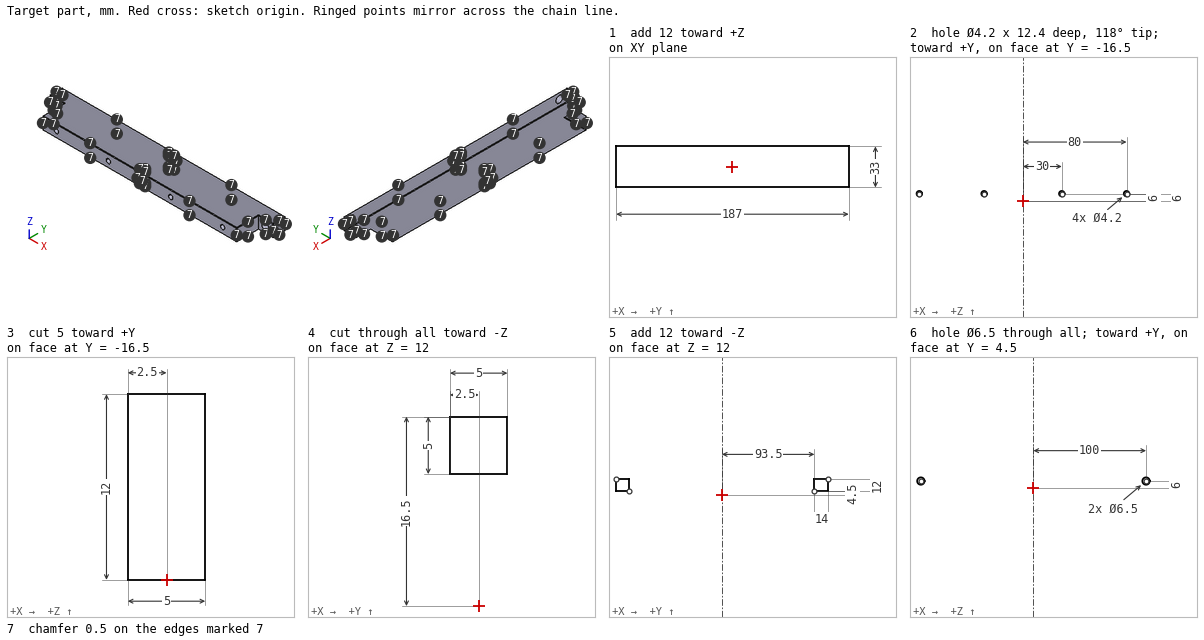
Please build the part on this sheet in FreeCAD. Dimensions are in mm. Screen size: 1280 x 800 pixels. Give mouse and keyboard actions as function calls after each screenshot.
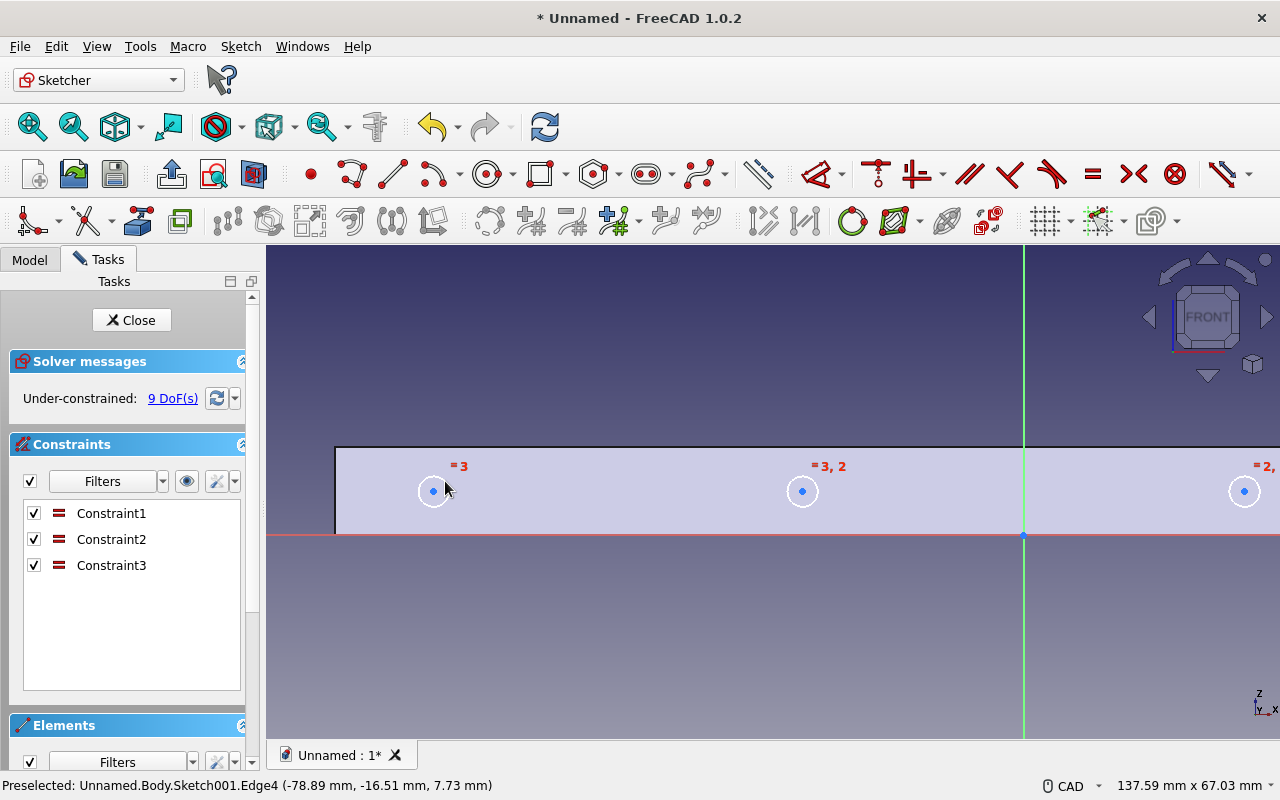
scroll(444, 481, down, 4)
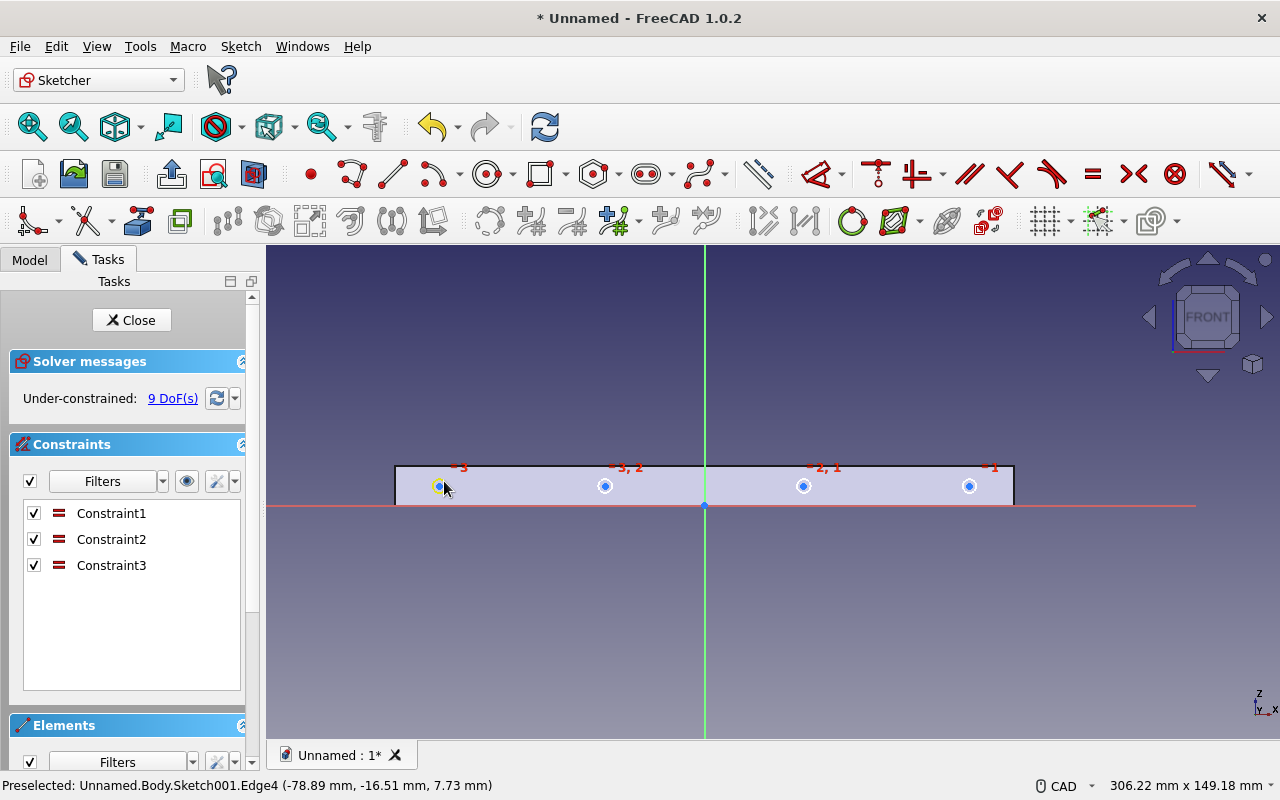
click(804, 486)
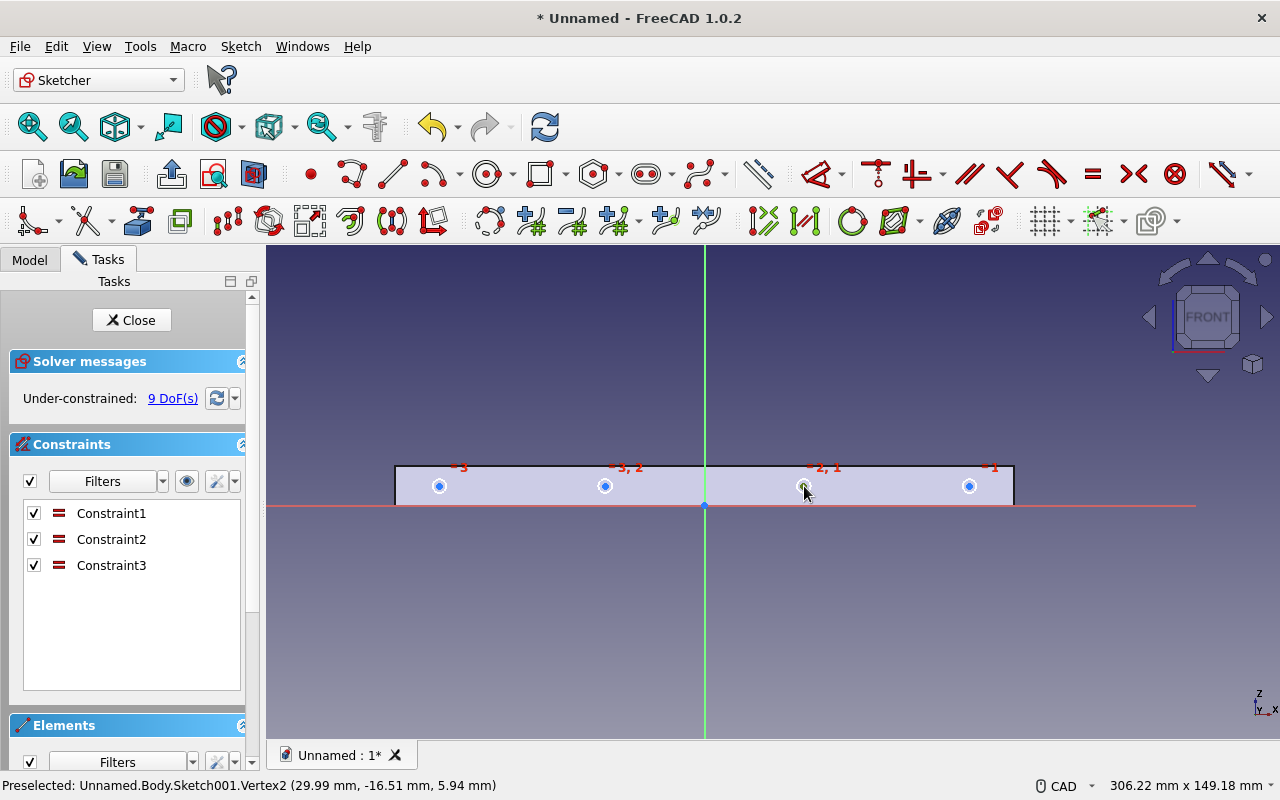
click(605, 486)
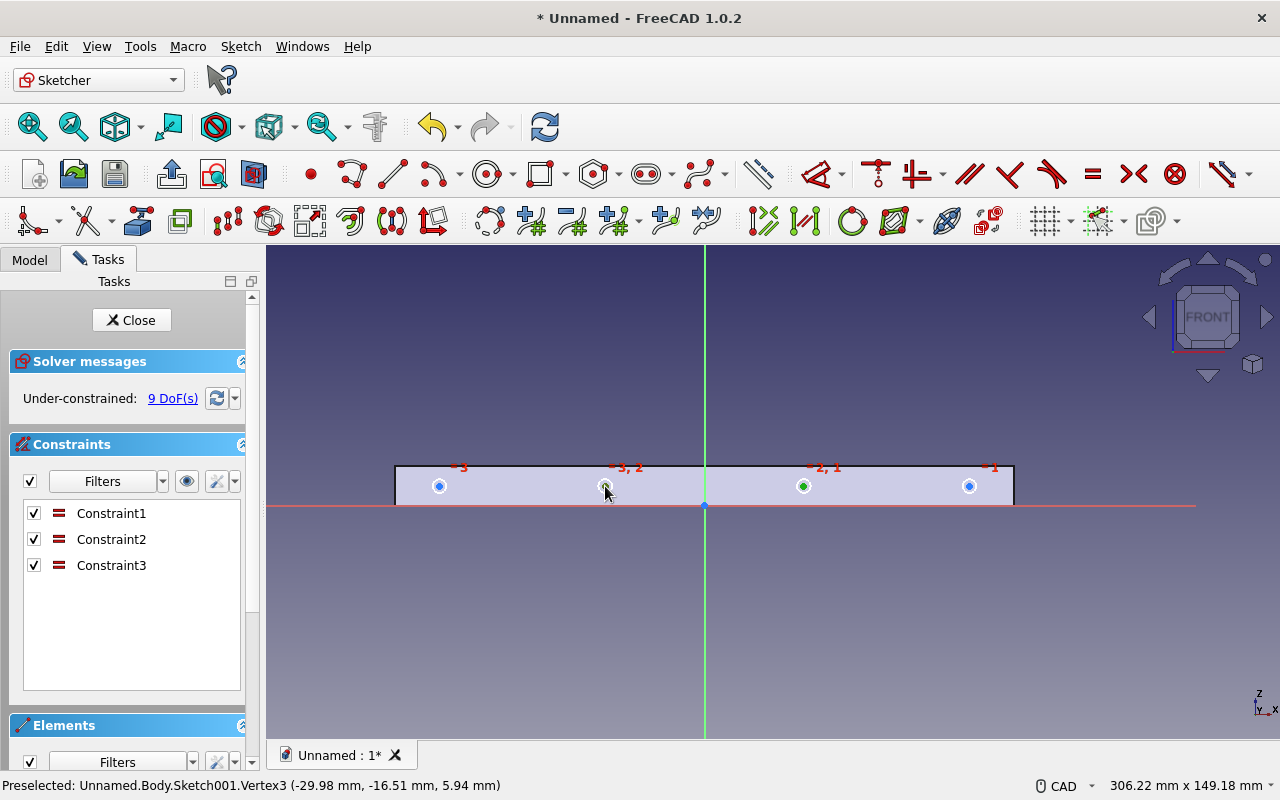
click(705, 680)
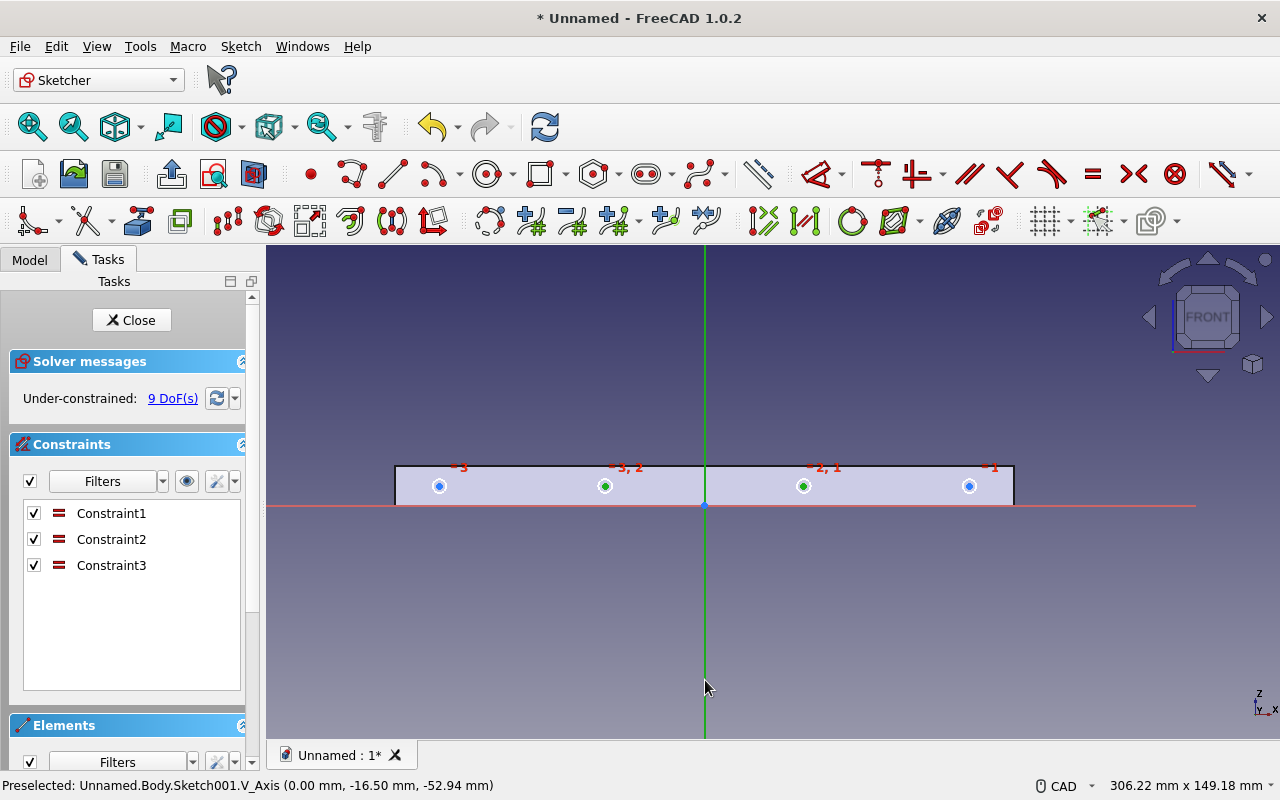
key(s)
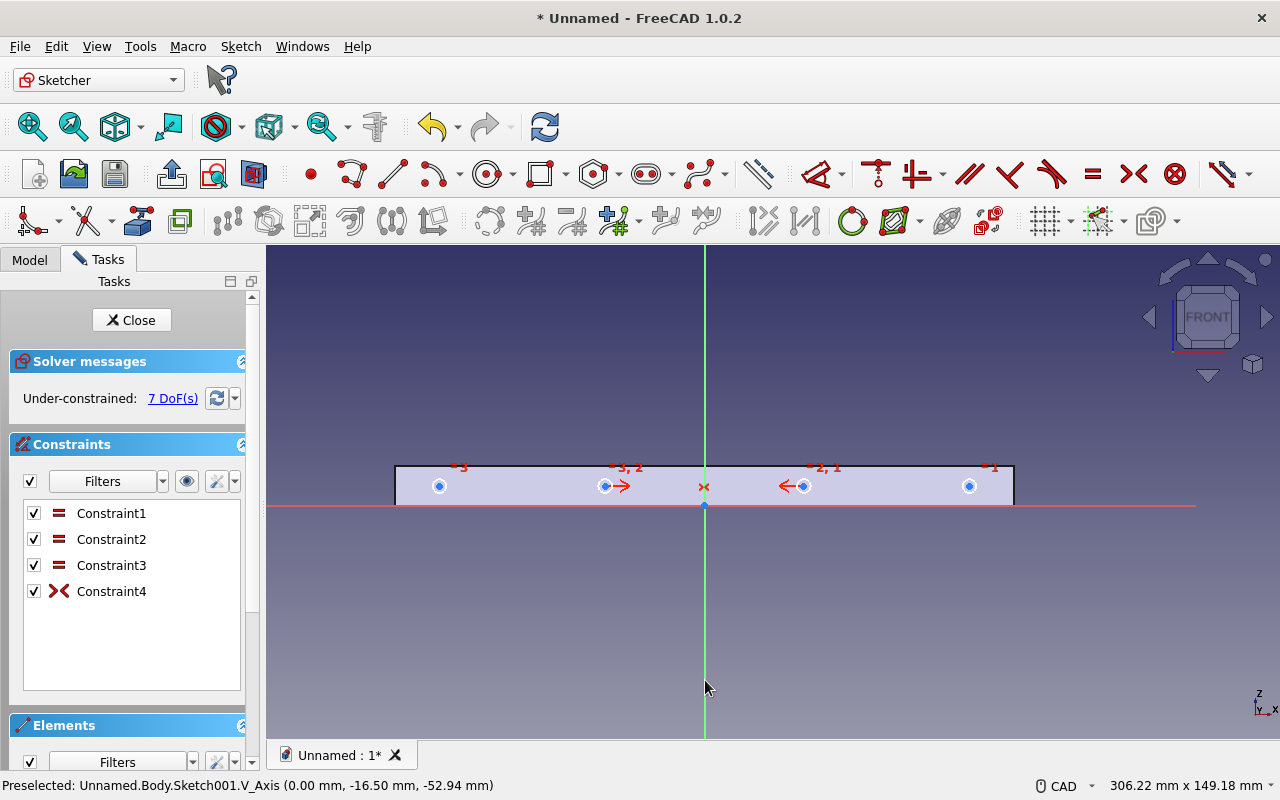
click(969, 486)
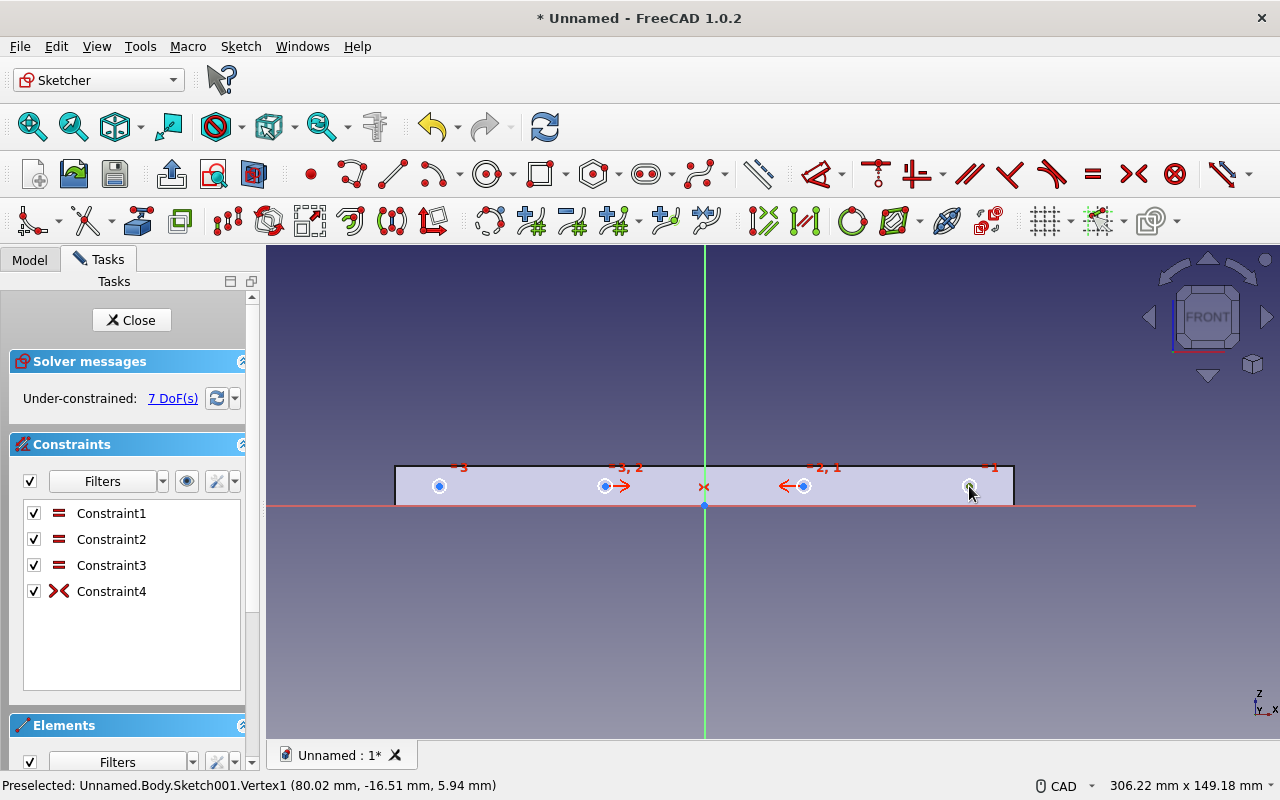
click(440, 486)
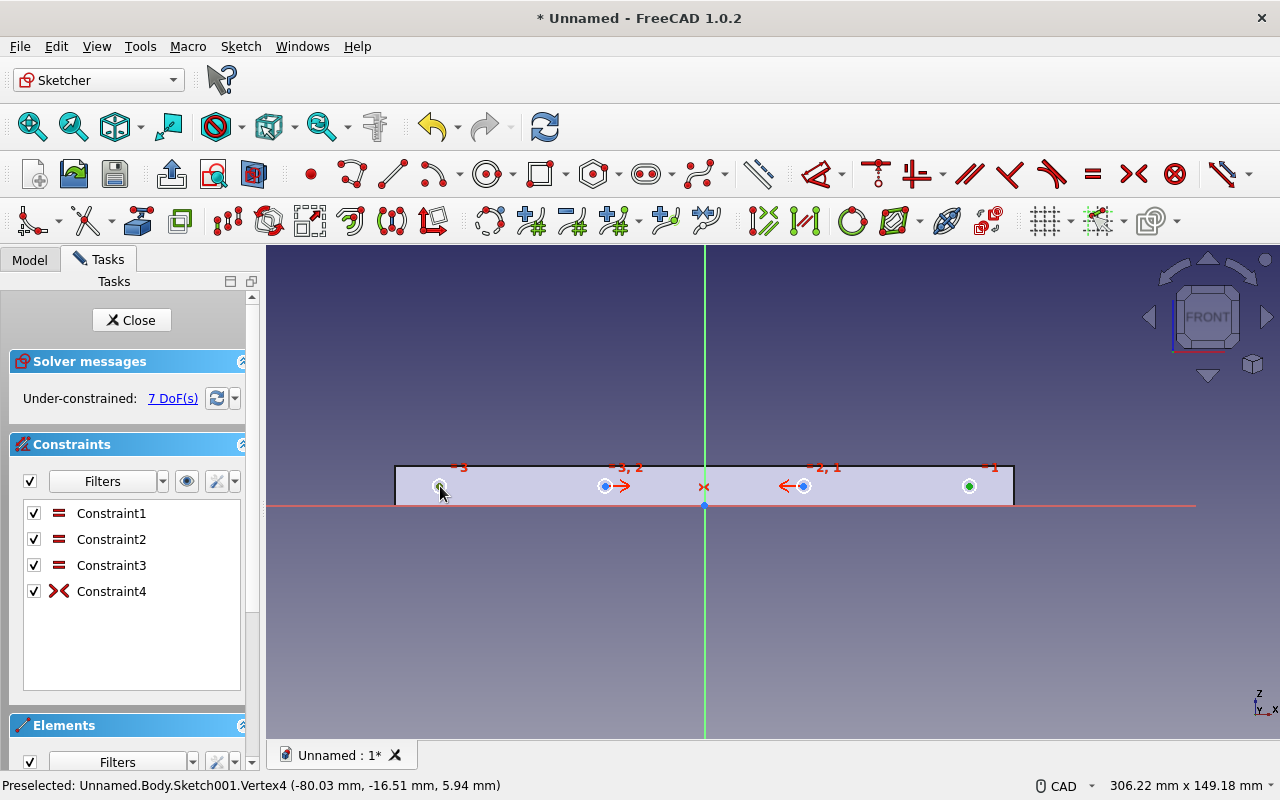
click(705, 680)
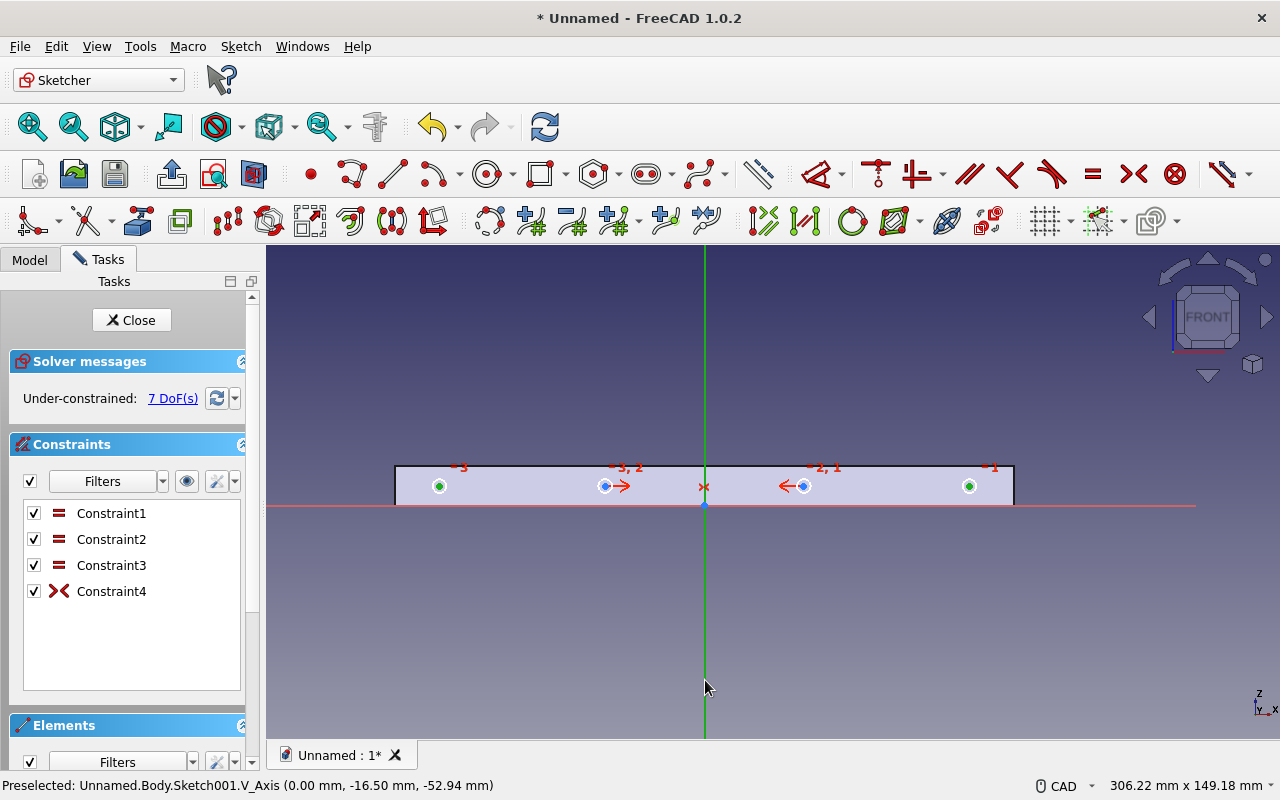
key(s)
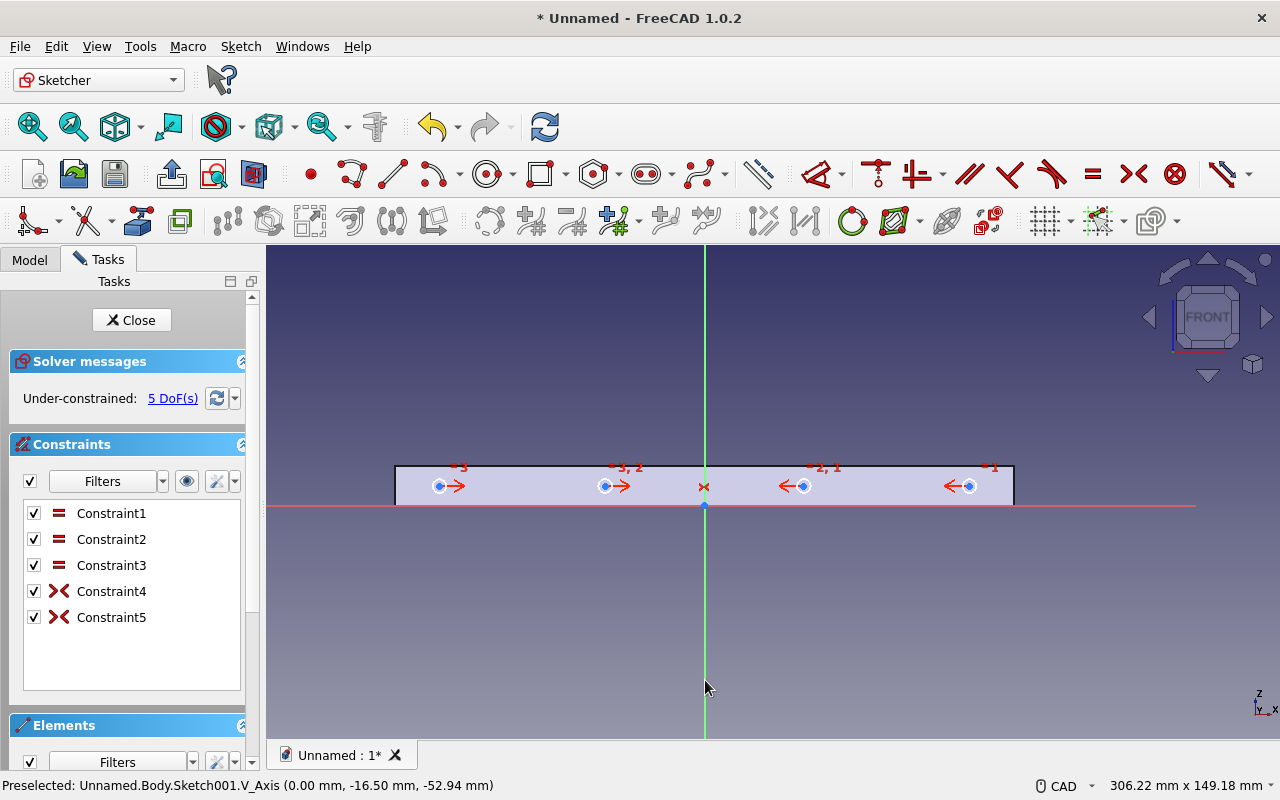
key(d)